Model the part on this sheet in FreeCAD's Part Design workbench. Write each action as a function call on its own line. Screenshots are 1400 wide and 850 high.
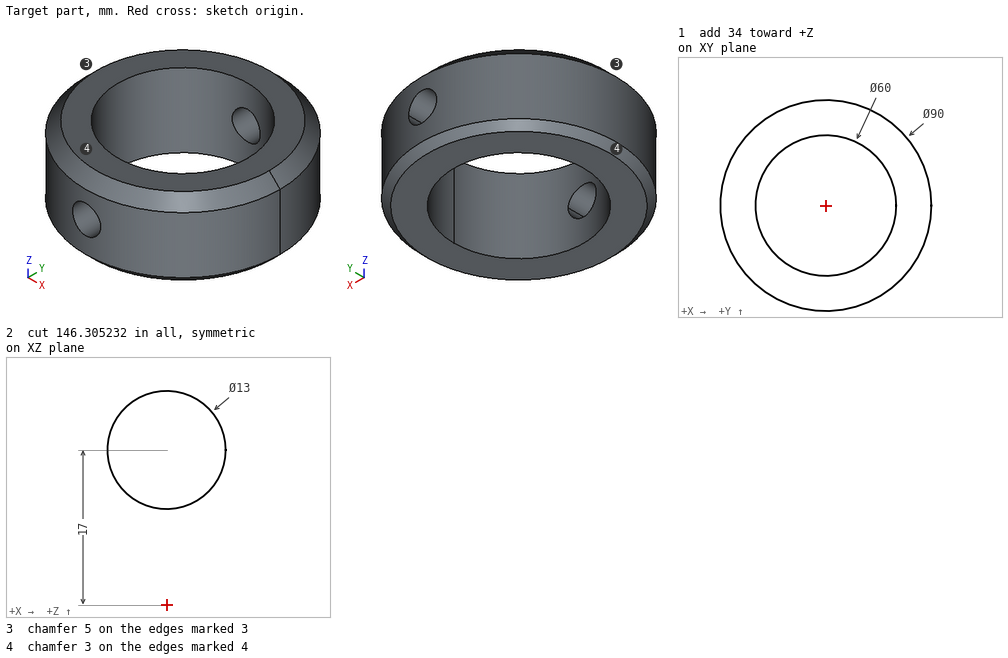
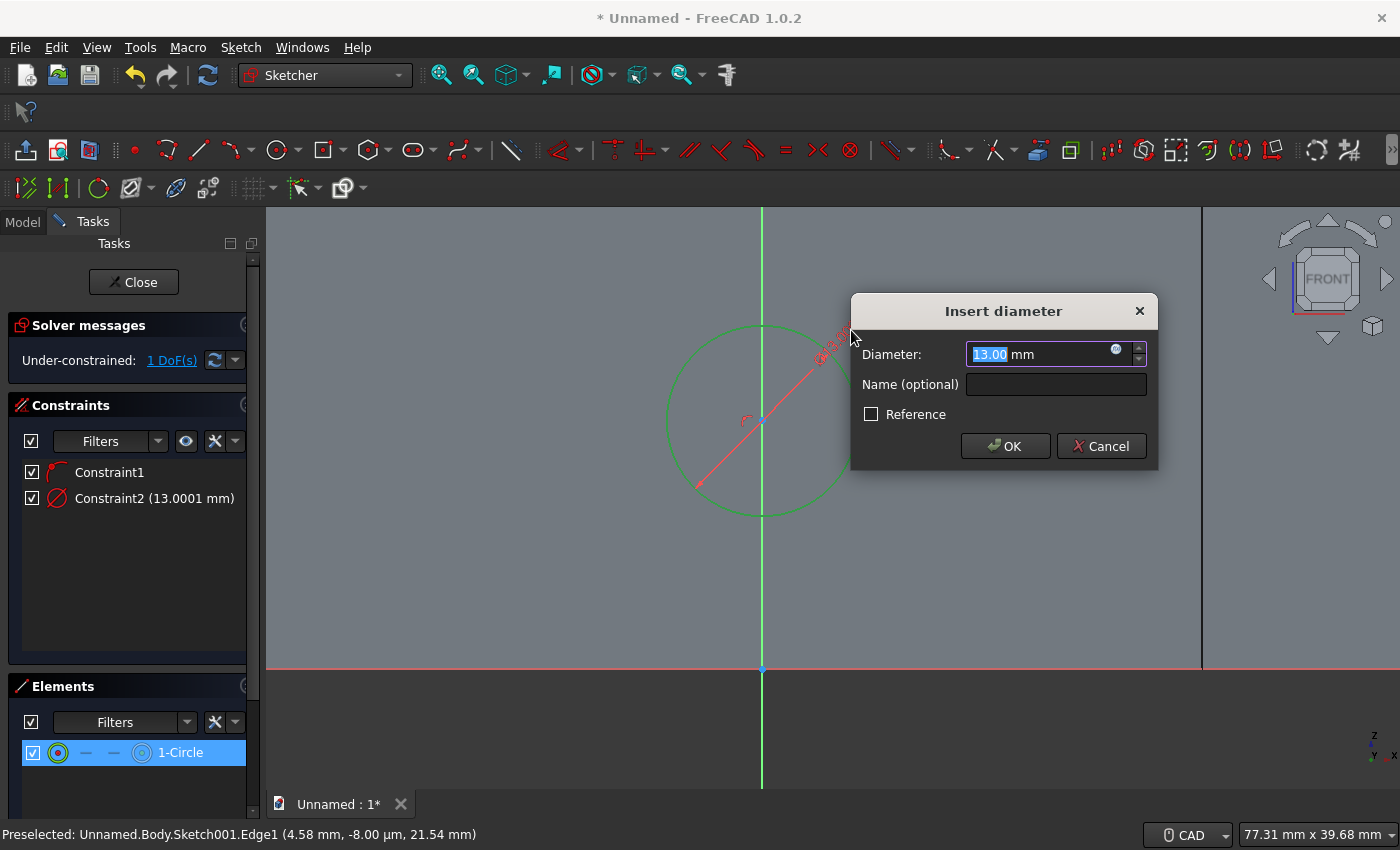
text(13)
key(Return)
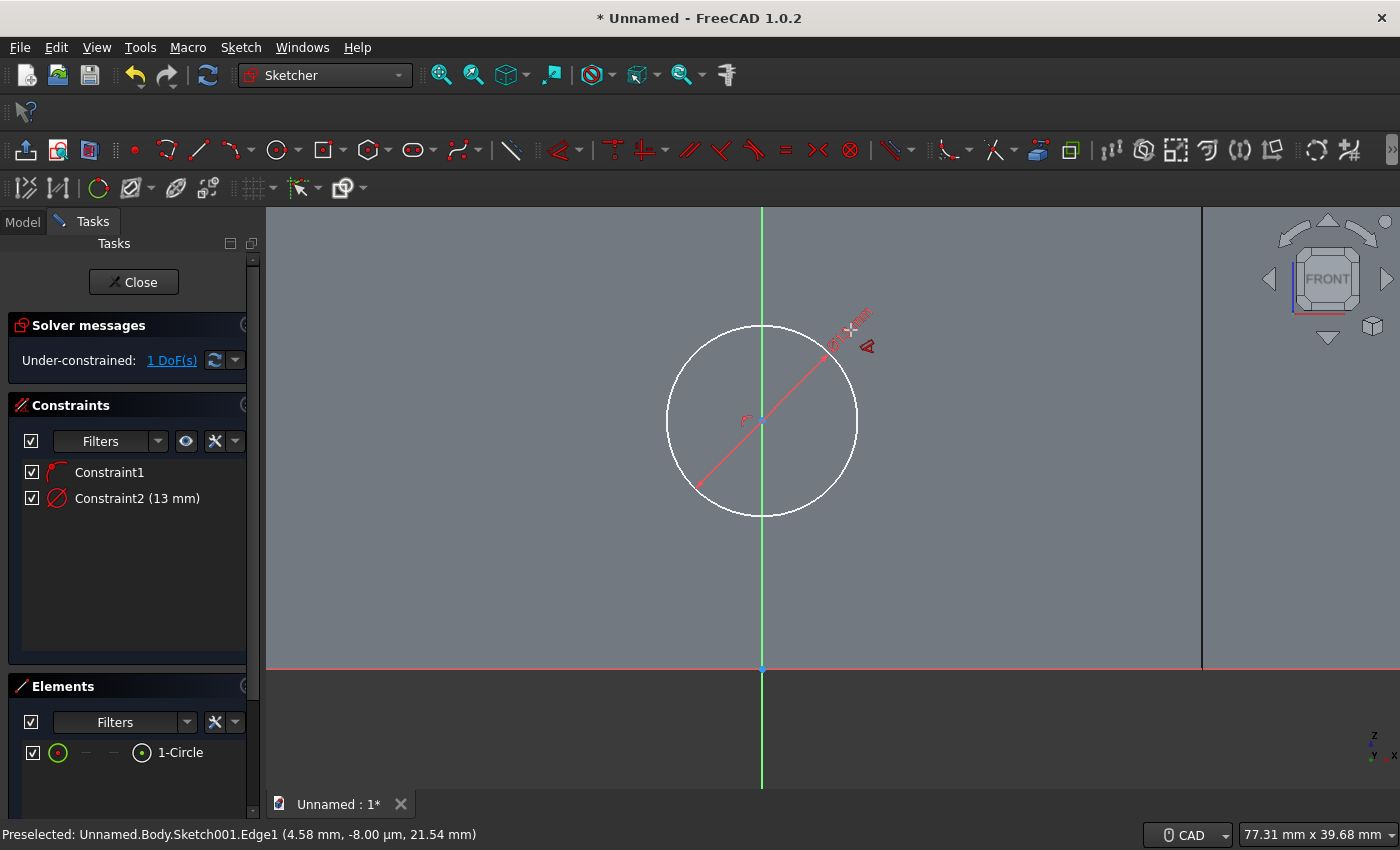
click(762, 421)
click(796, 545)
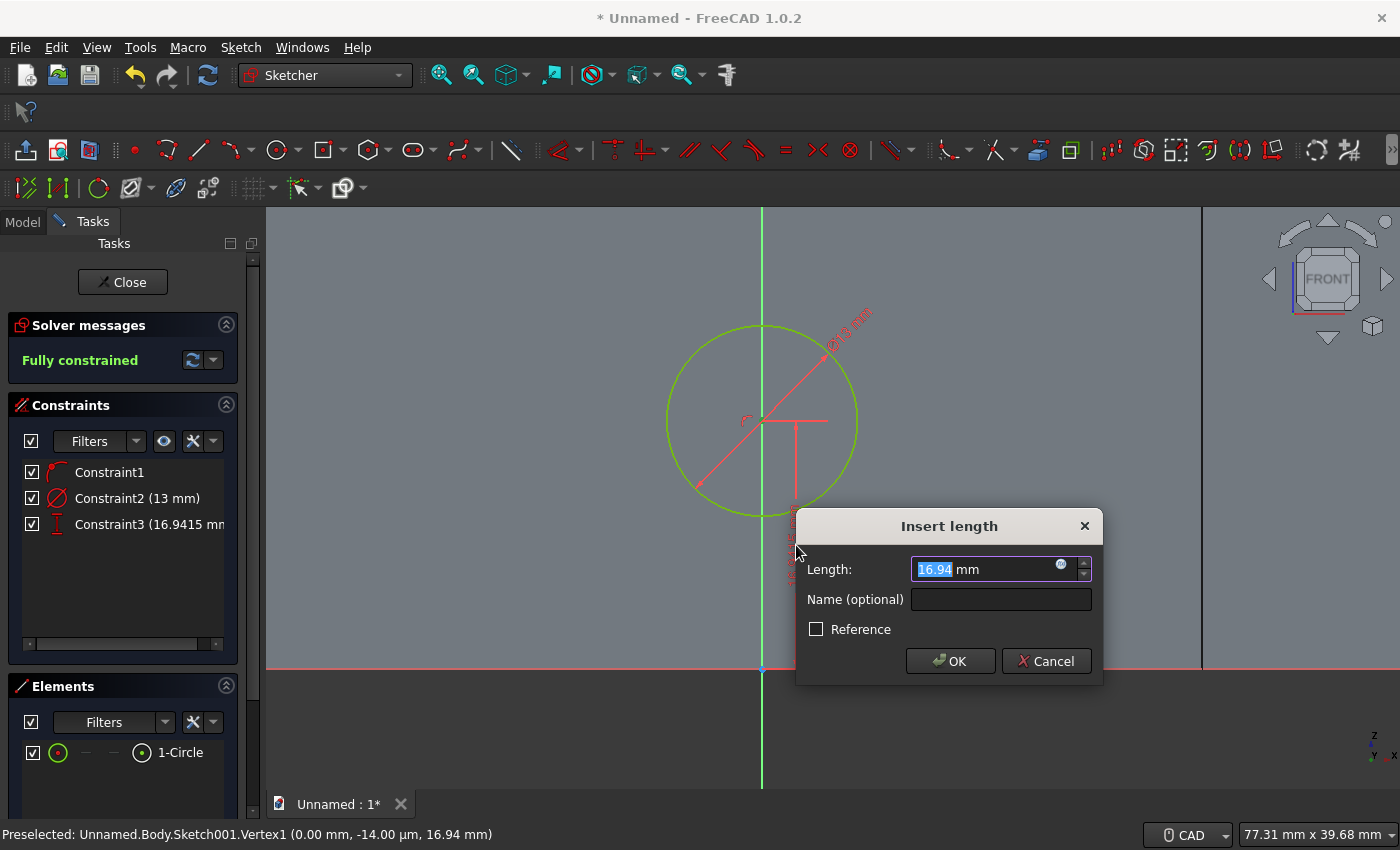
text(17)
key(Return)
key(Escape)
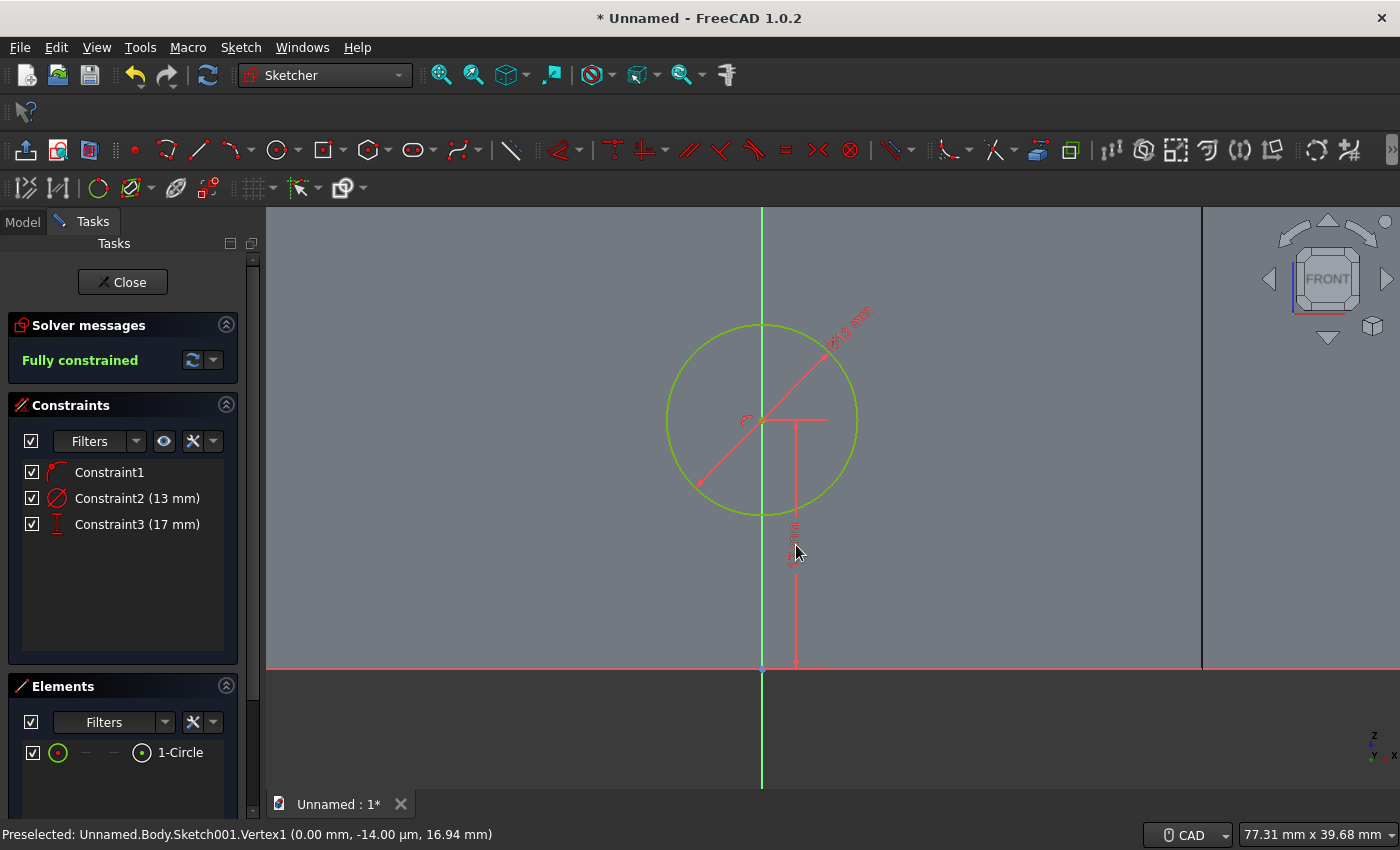
click(123, 282)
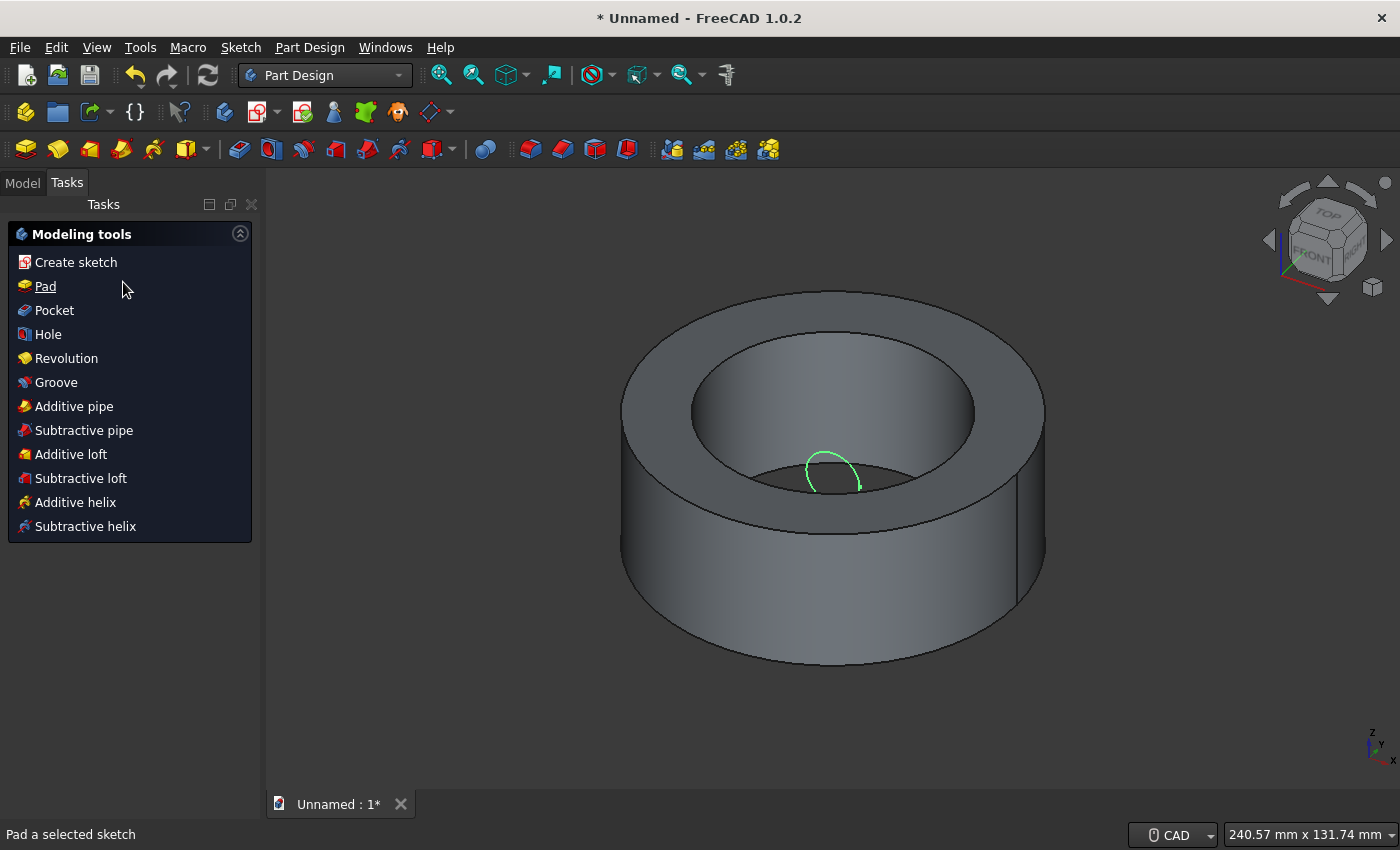
click(240, 150)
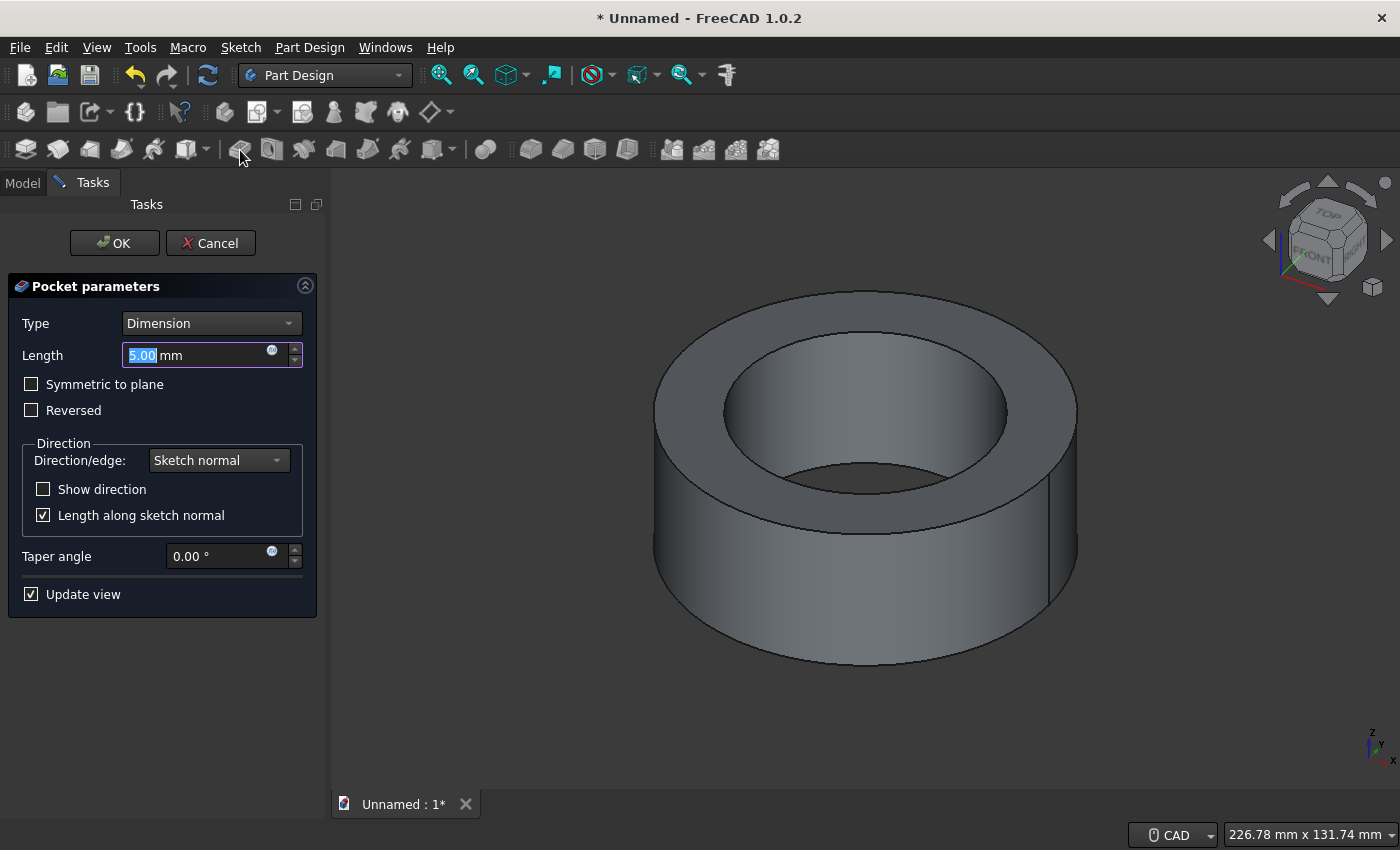
text(146.305232)
key(Tab)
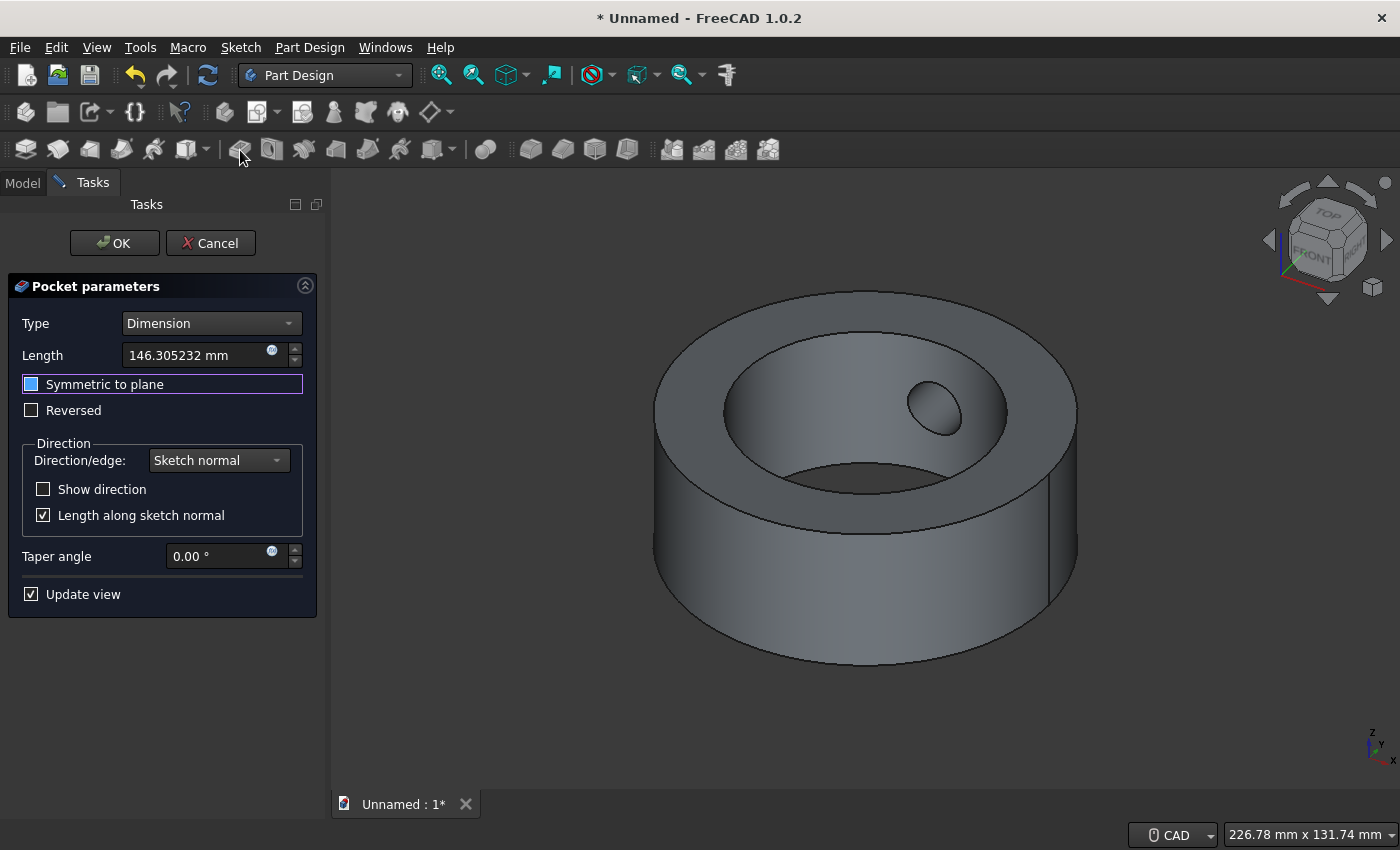
click(30, 384)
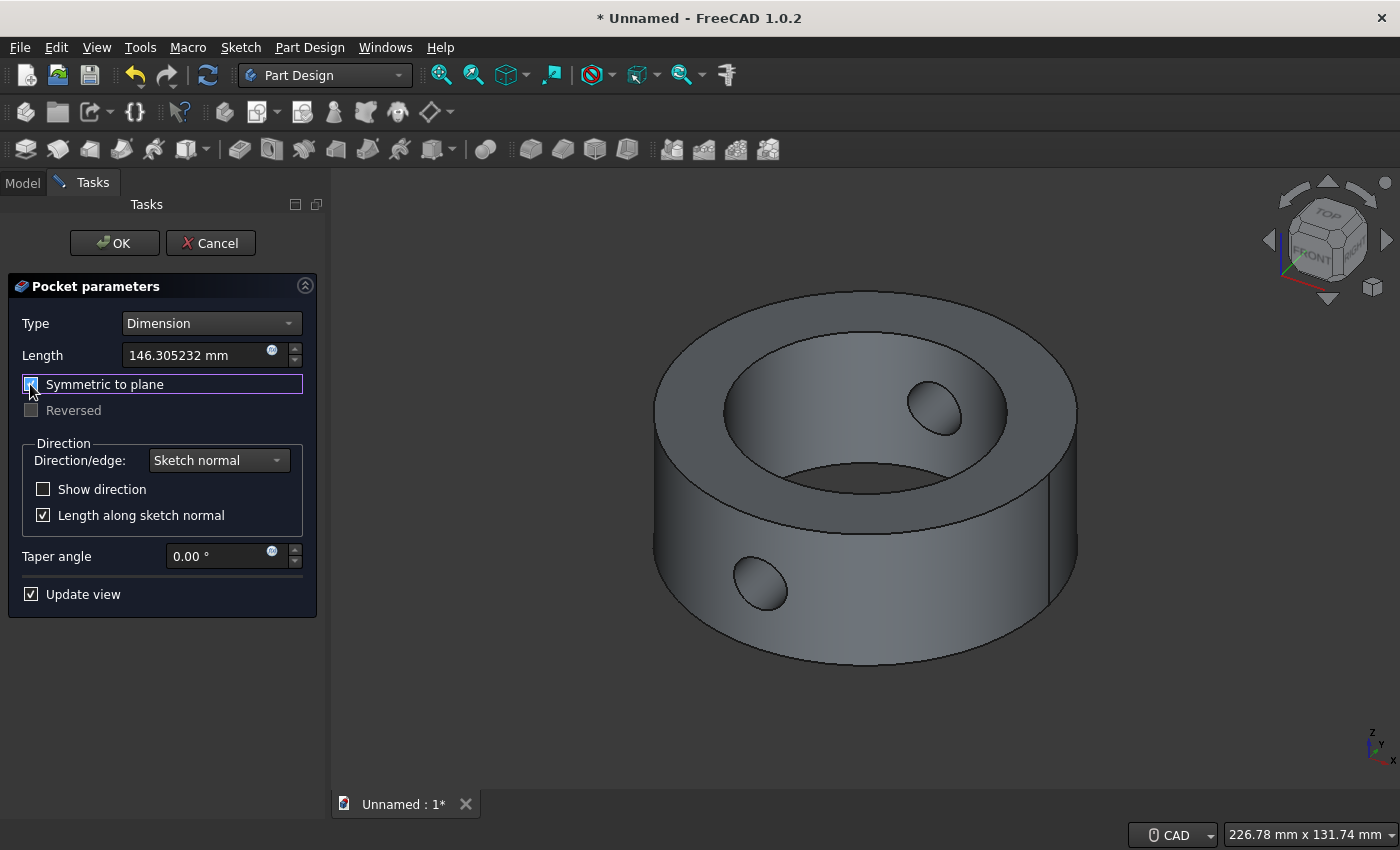
click(115, 243)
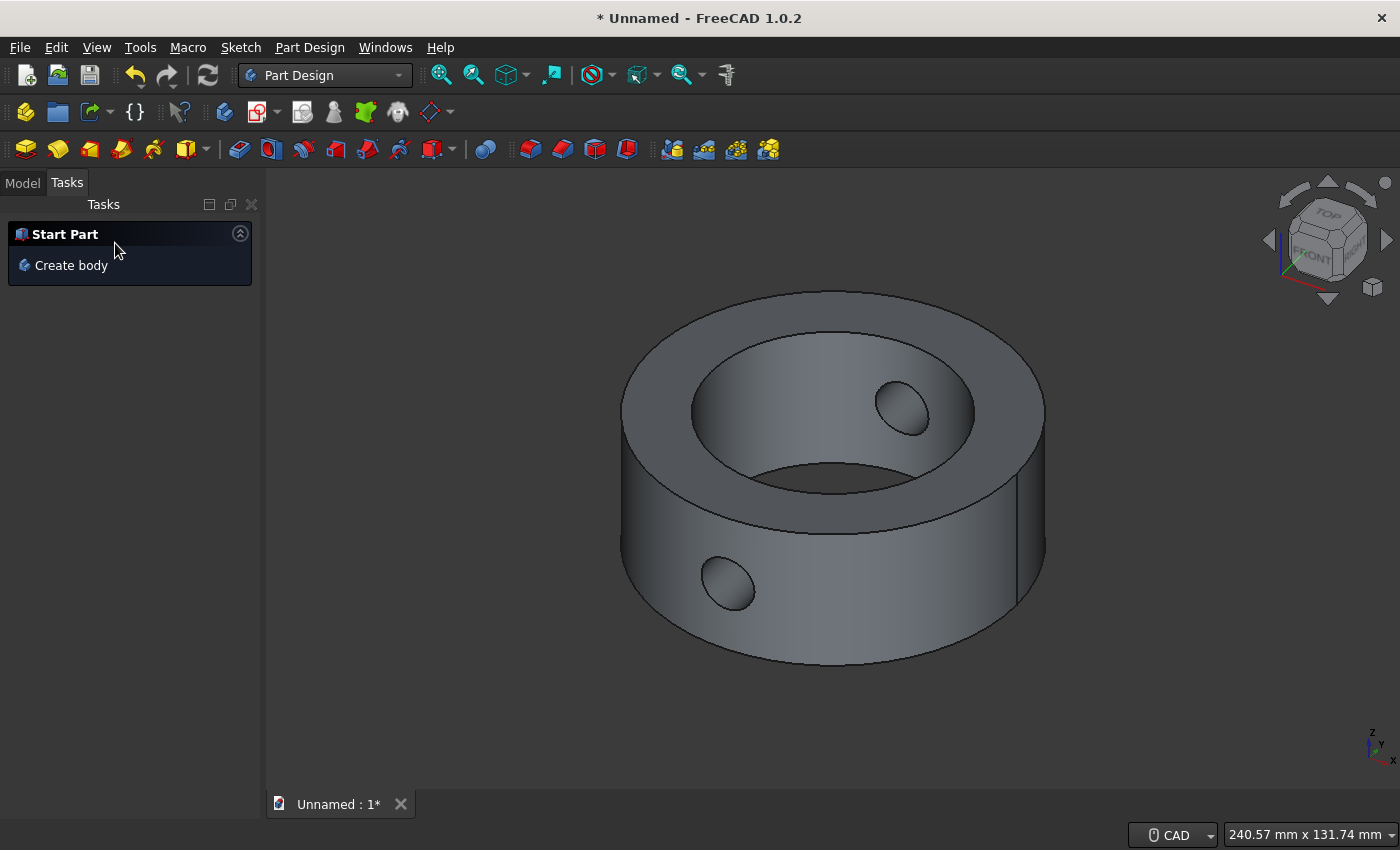
click(622, 425)